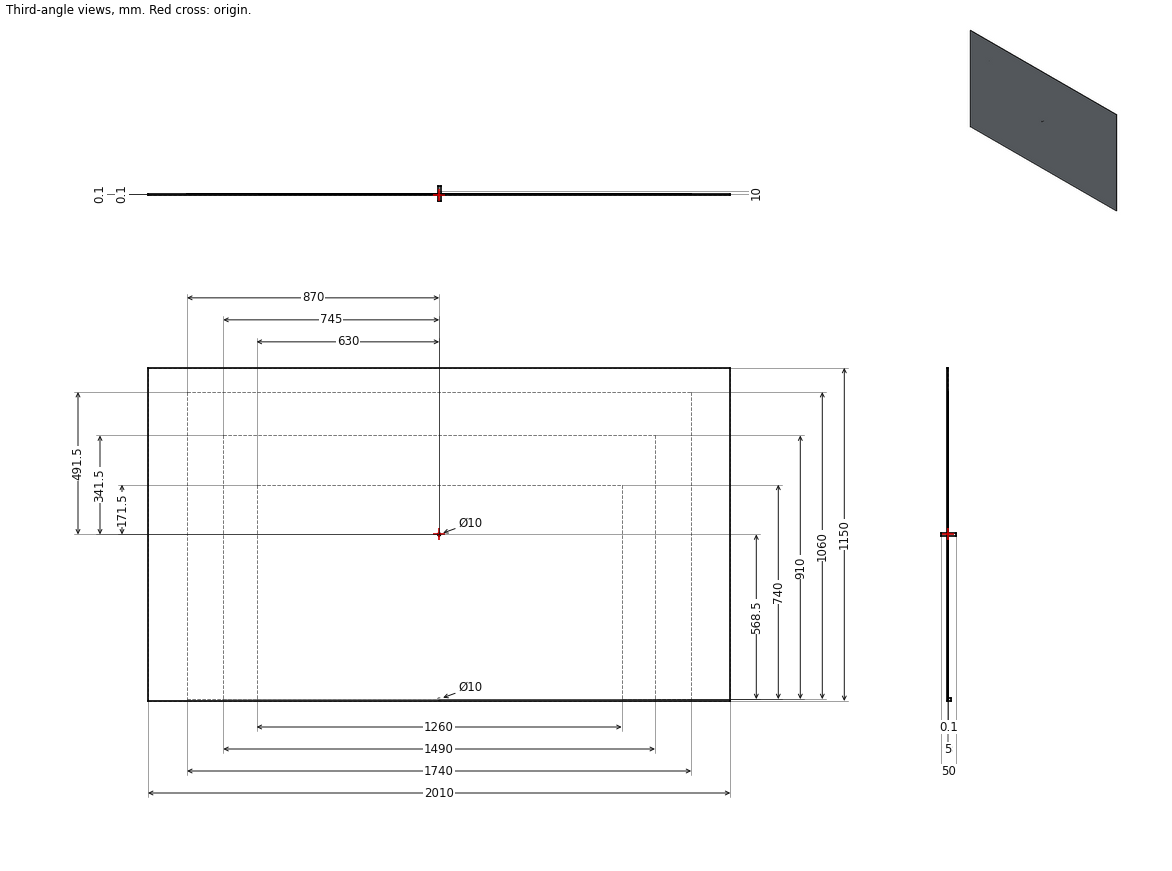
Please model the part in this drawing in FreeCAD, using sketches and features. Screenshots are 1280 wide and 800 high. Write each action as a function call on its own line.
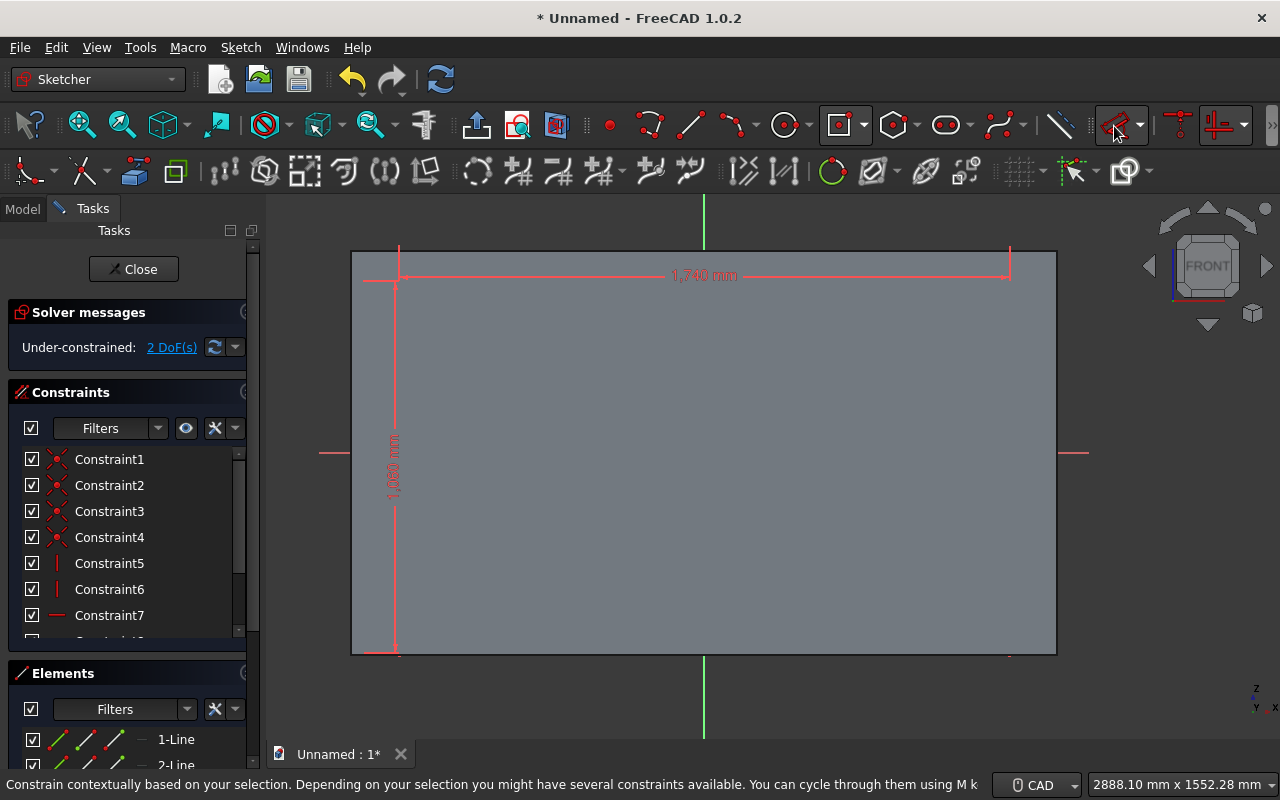
click(399, 281)
click(552, 247)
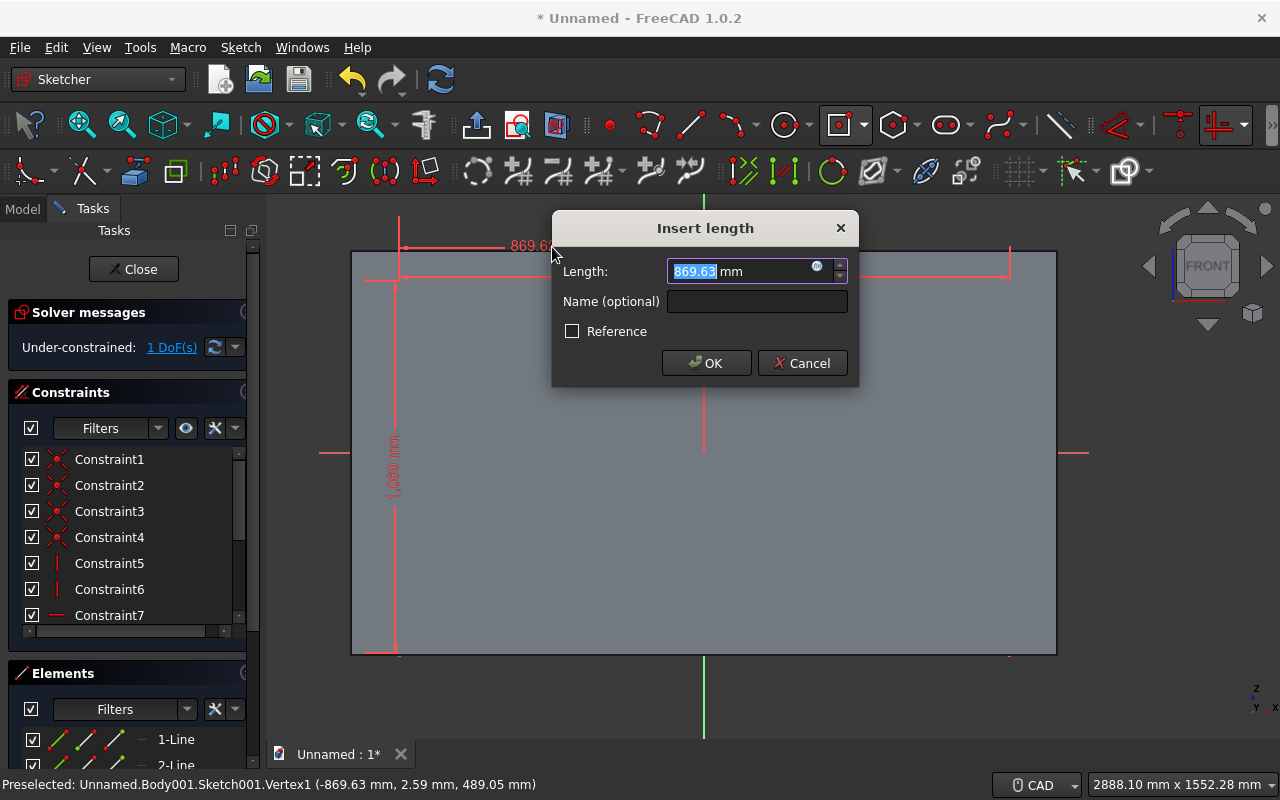
text(870)
key(Return)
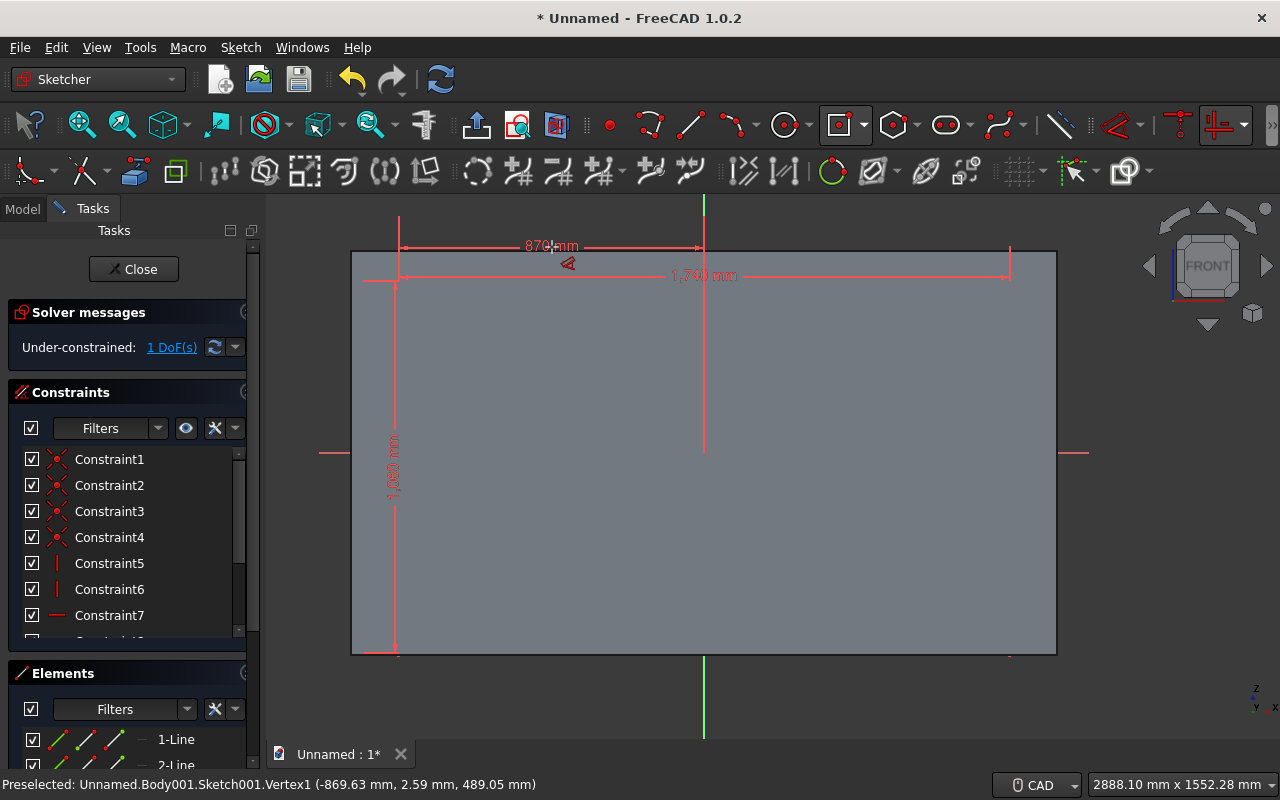
click(399, 281)
click(365, 367)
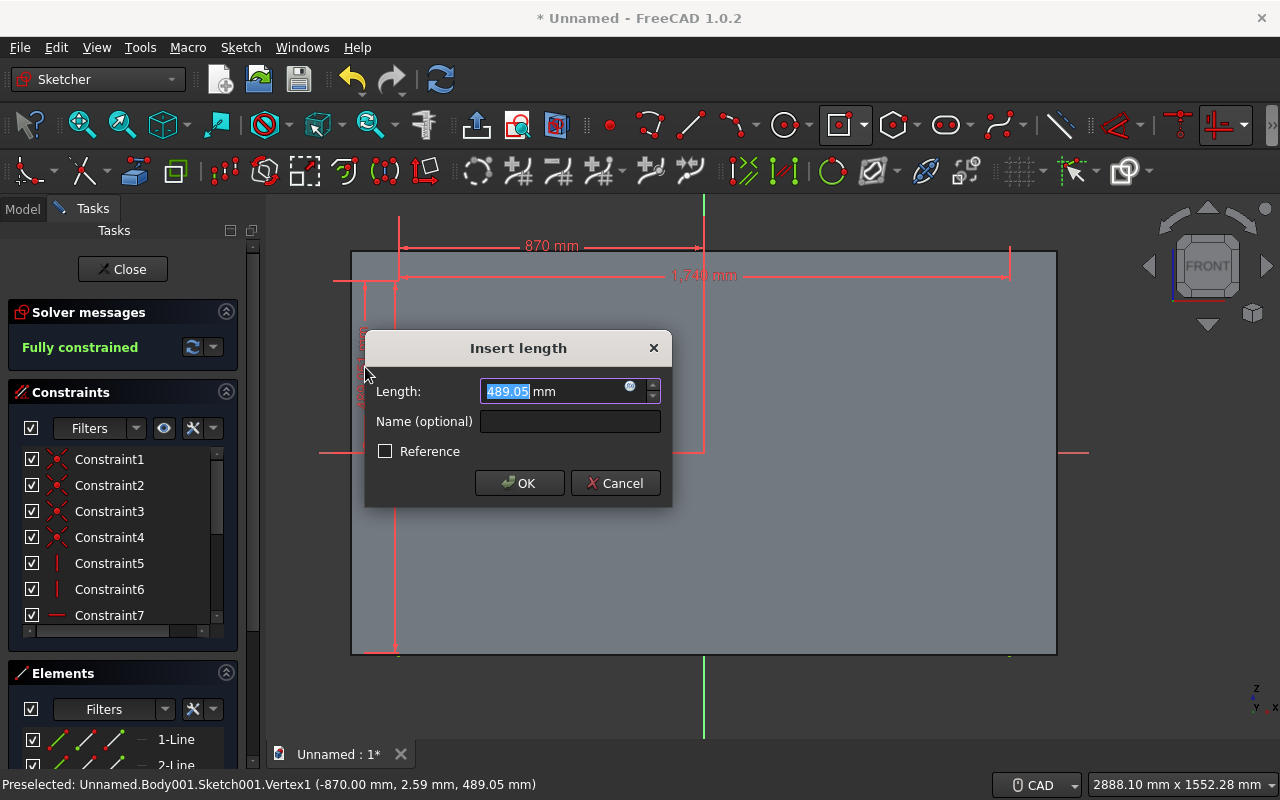
text(491.5)
key(Return)
key(Escape)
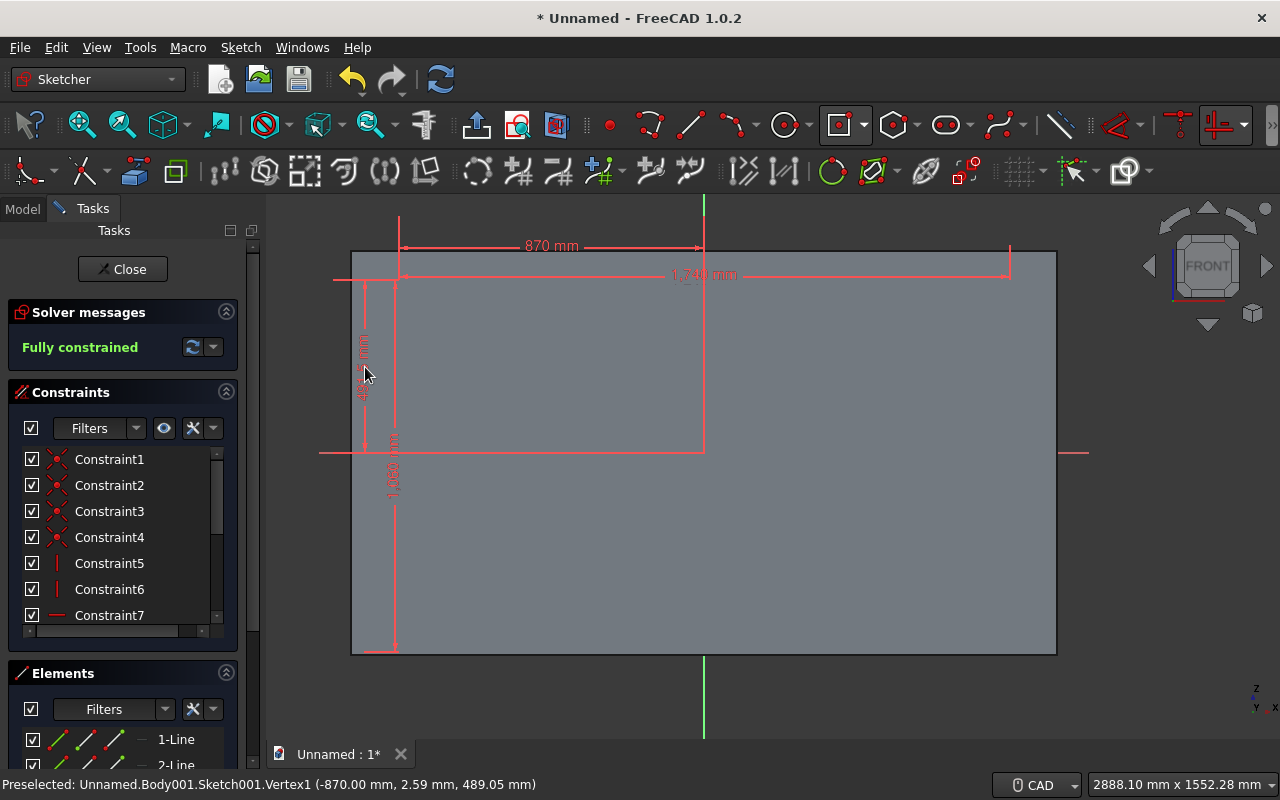
click(123, 269)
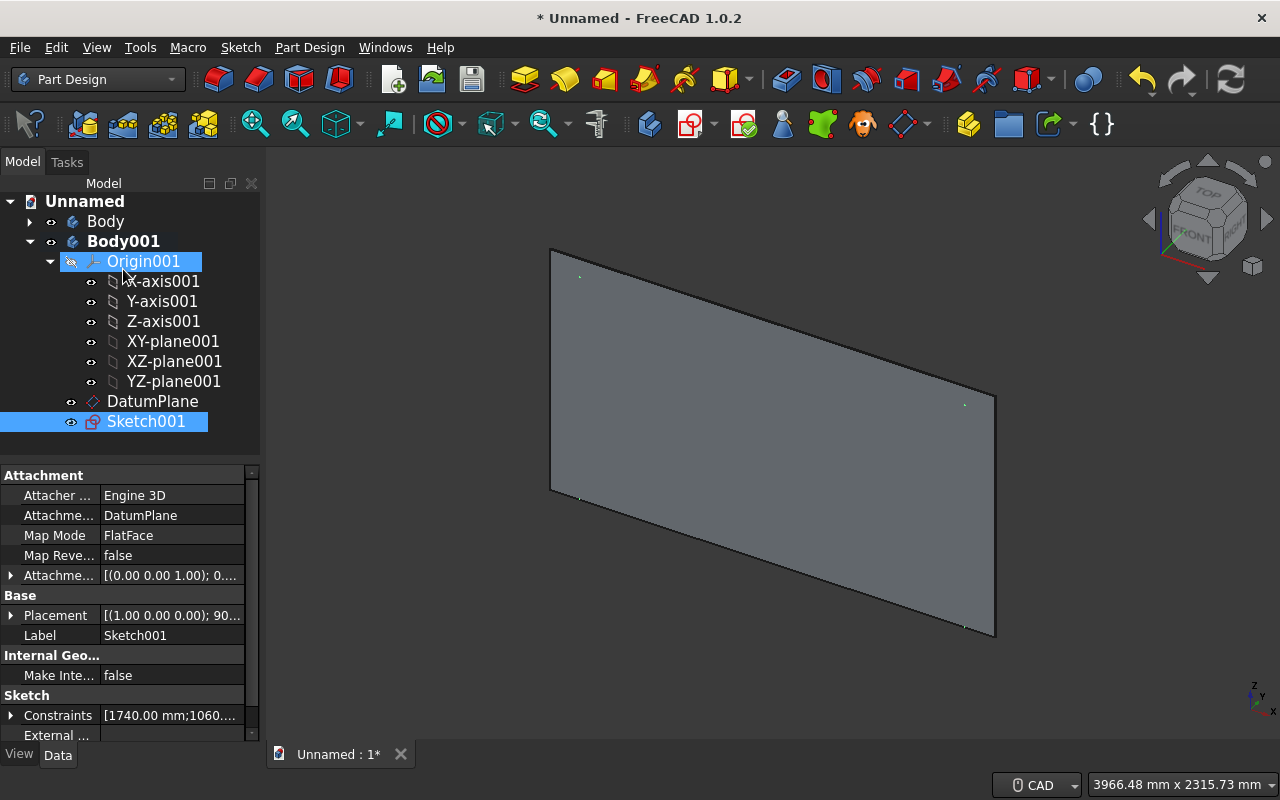
click(526, 80)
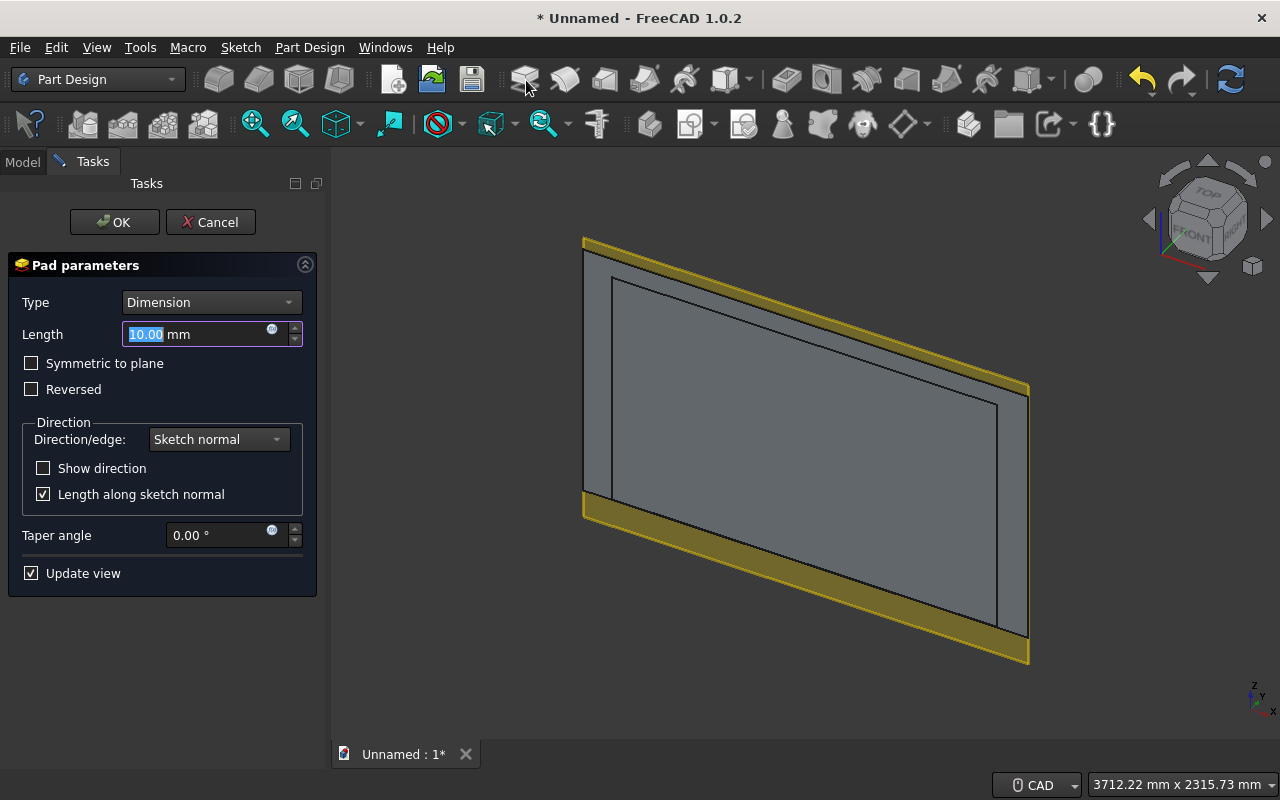
text(0.1)
key(Tab)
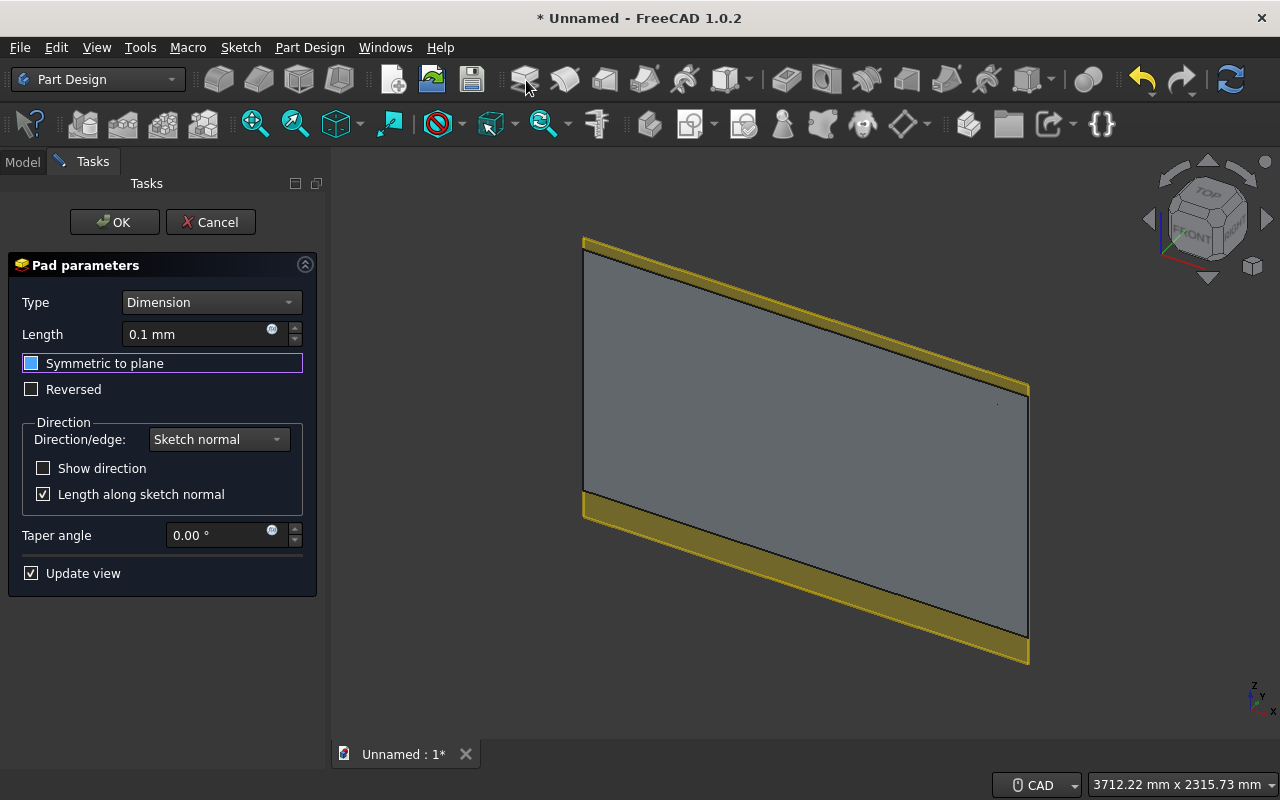
click(30, 389)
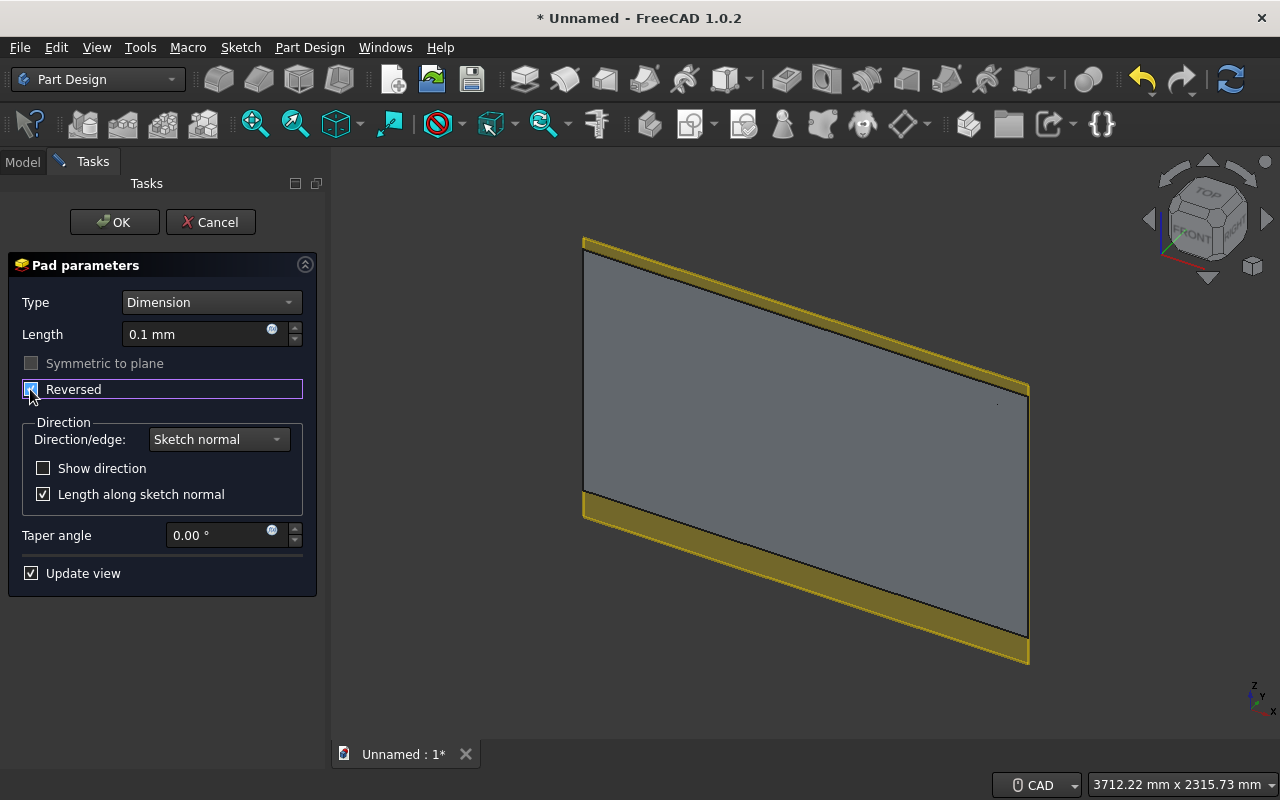
click(115, 222)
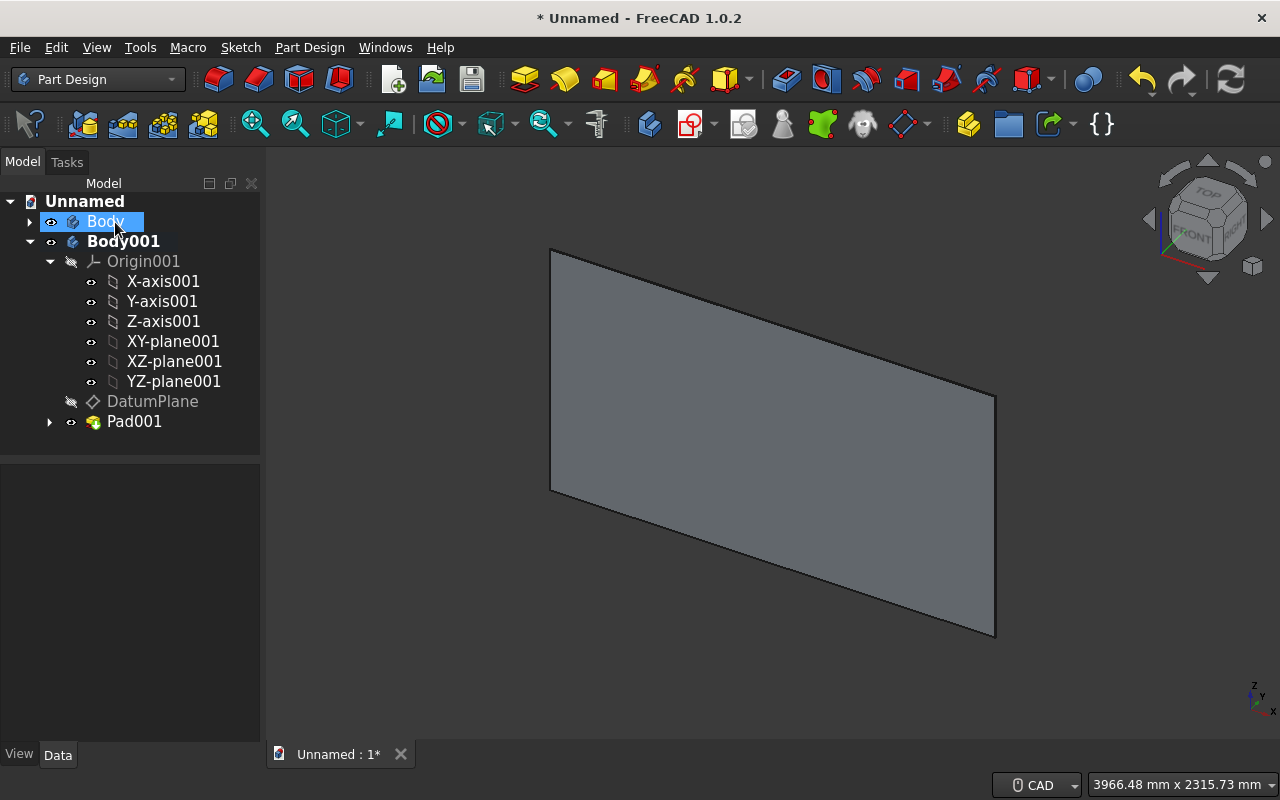
click(650, 124)